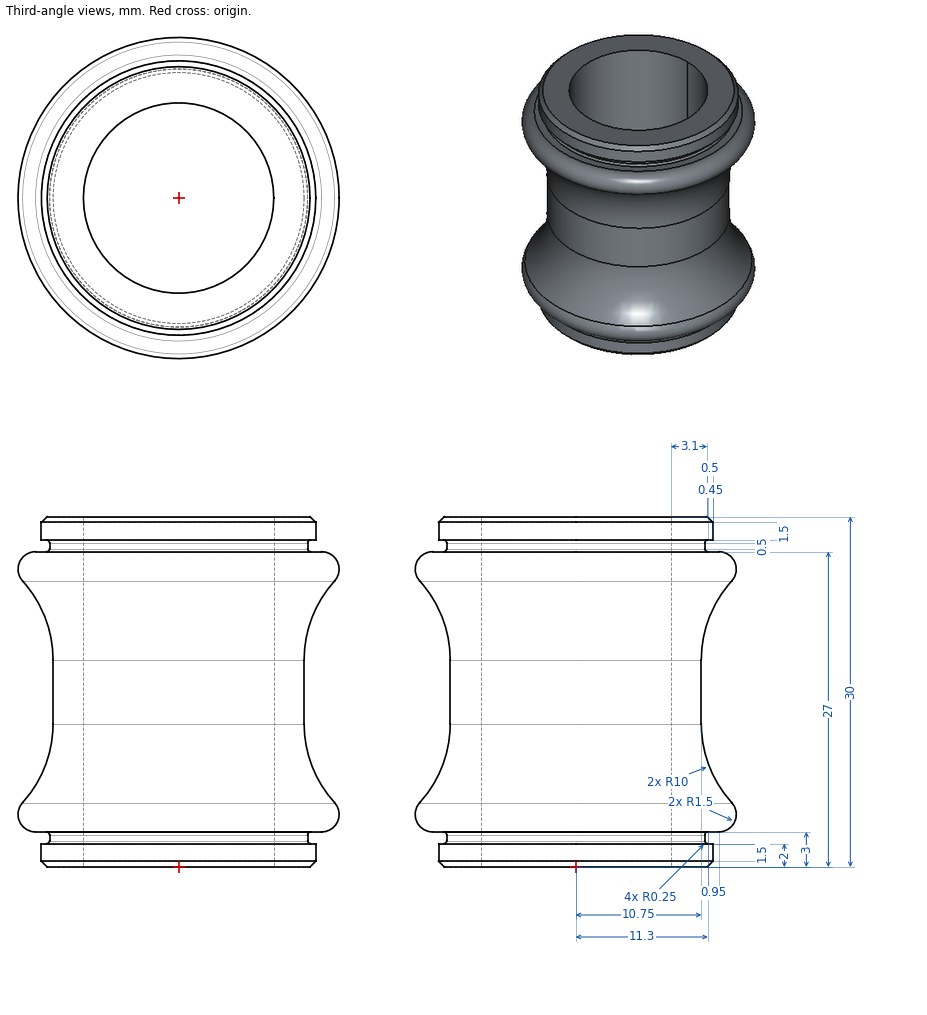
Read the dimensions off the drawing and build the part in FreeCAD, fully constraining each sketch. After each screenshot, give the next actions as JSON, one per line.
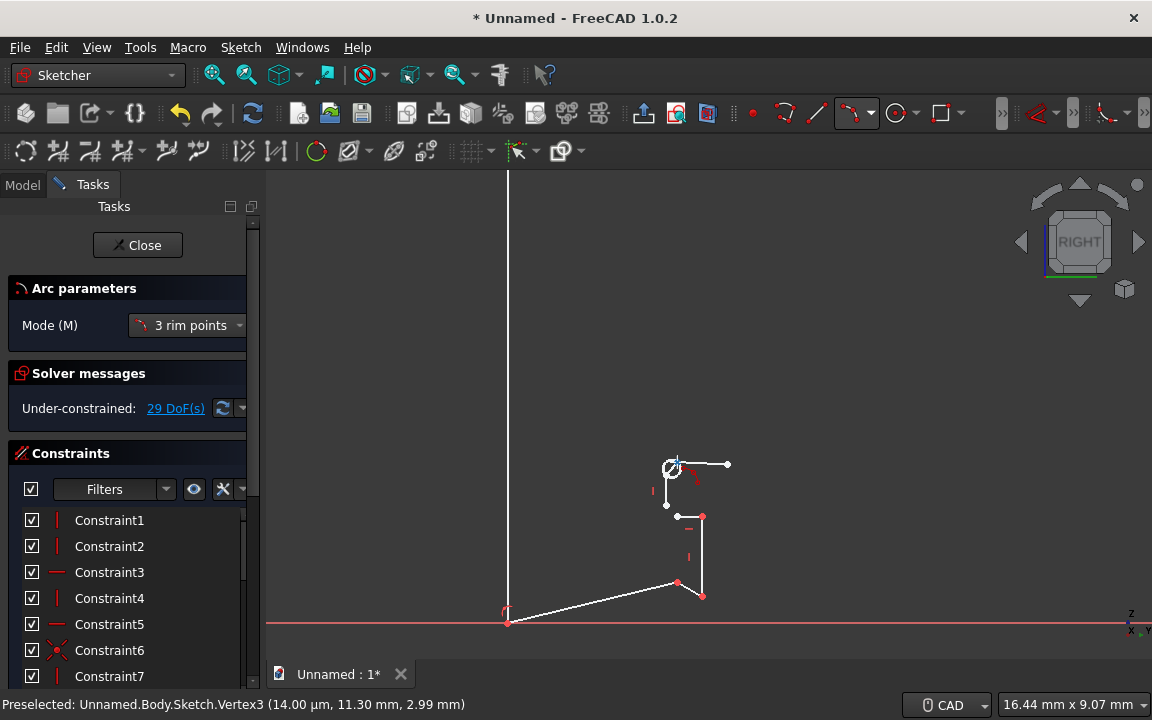
{"action": "scroll", "coordinate": [668, 465], "scroll_direction": "up", "scroll_amount": 7}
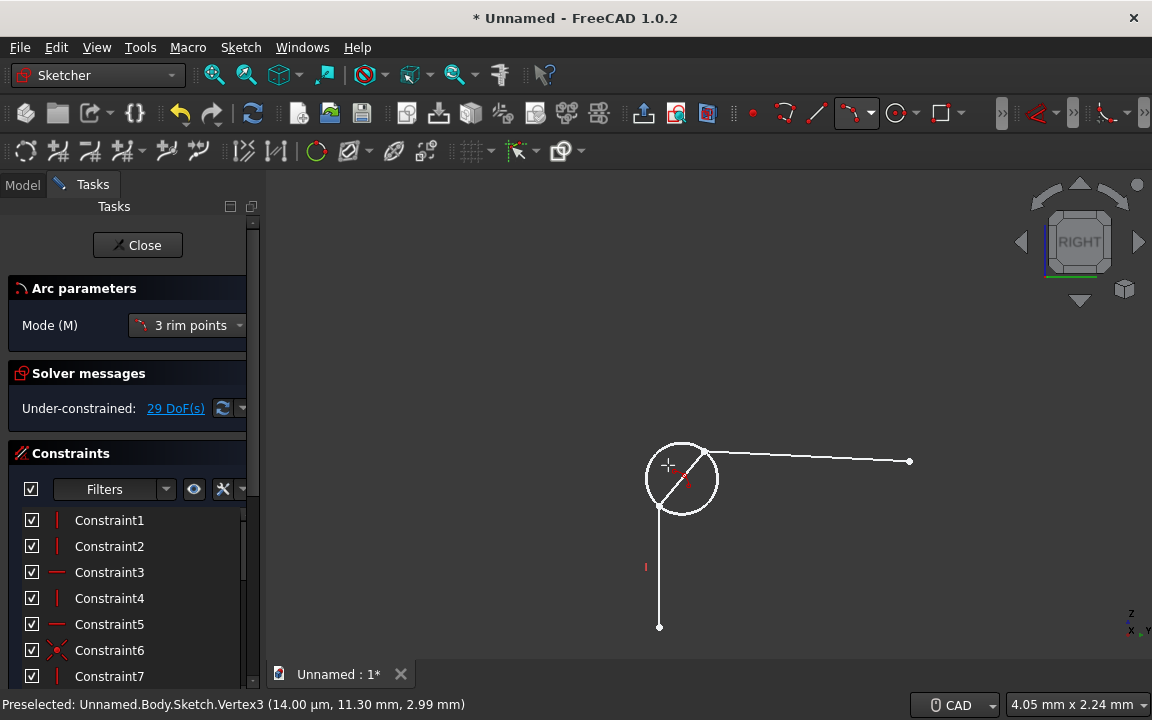
{"action": "left_click", "coordinate": [667, 464]}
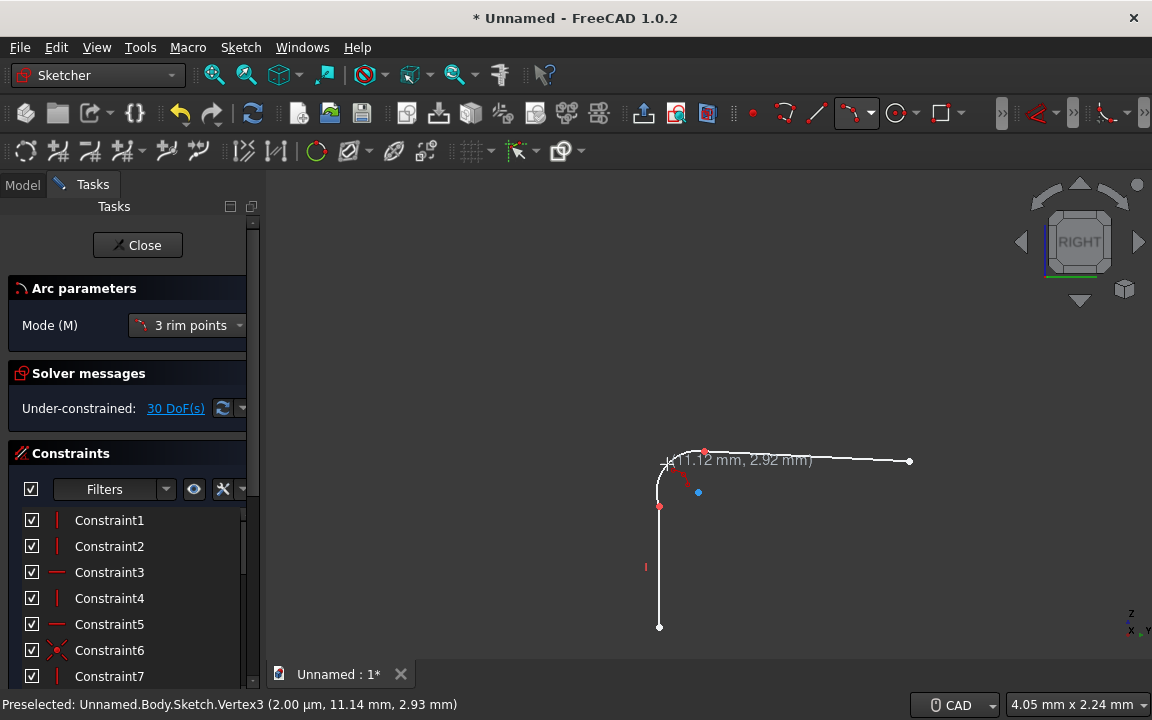
{"action": "scroll", "coordinate": [689, 550], "scroll_direction": "down", "scroll_amount": 15}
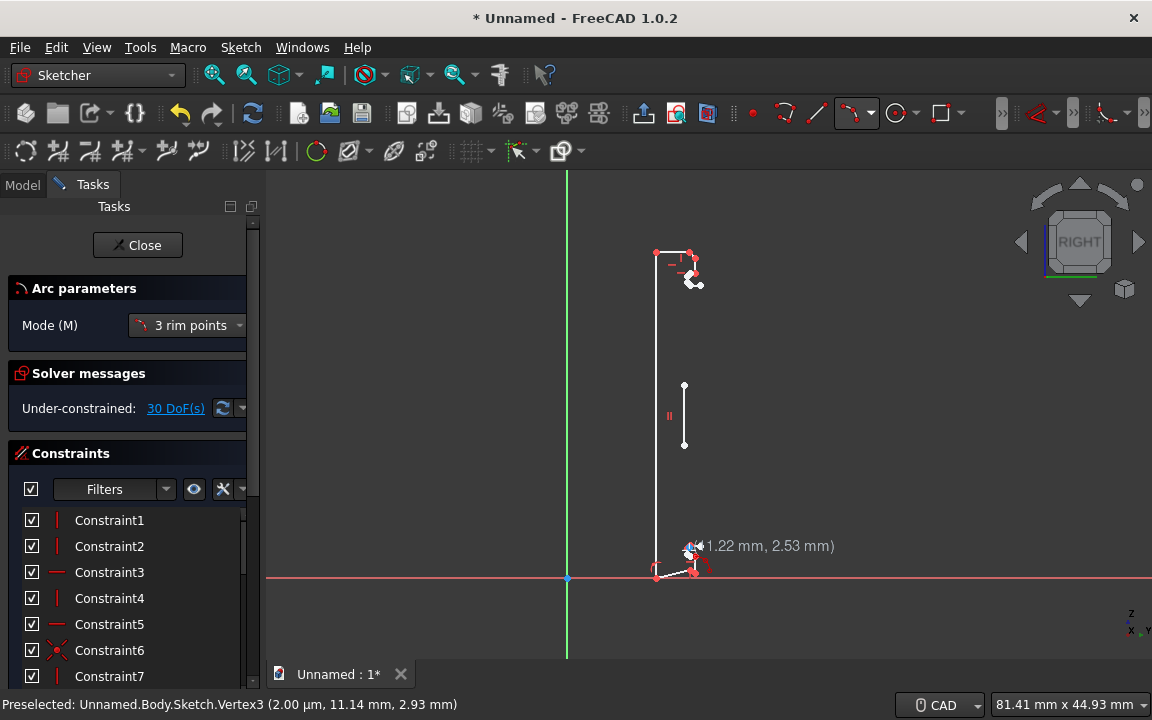
{"action": "scroll", "coordinate": [701, 546], "scroll_direction": "up", "scroll_amount": 6}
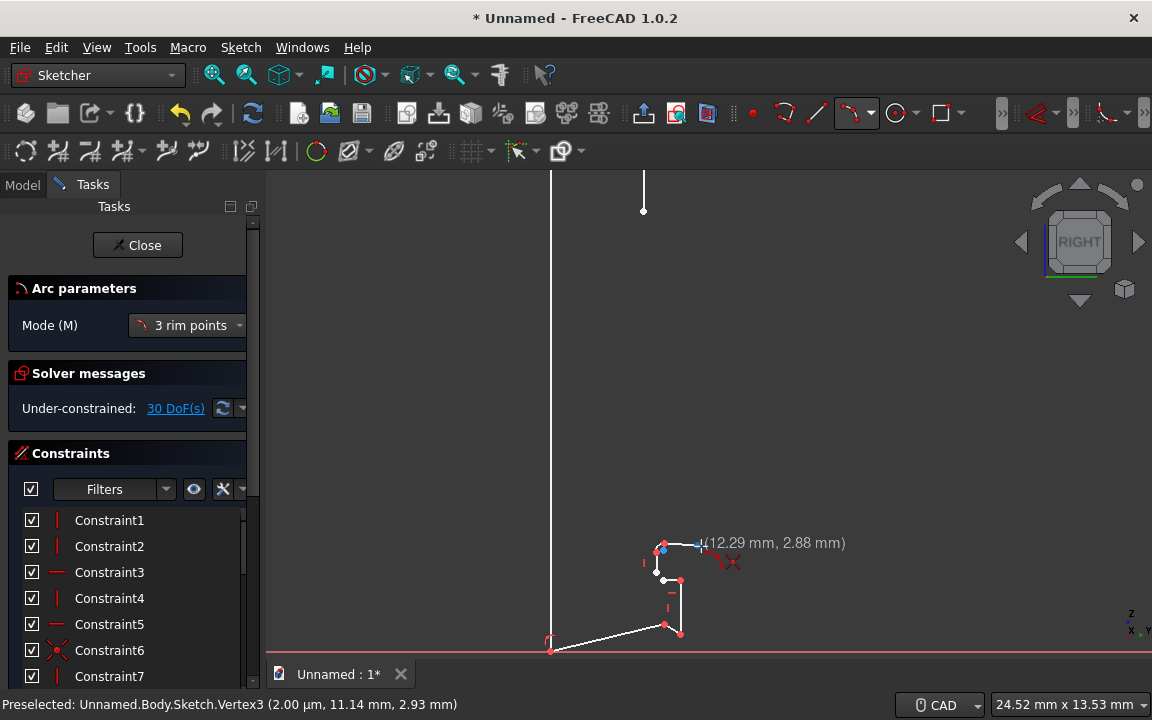
{"action": "left_click", "coordinate": [698, 545]}
{"action": "left_click", "coordinate": [739, 452]}
{"action": "left_click", "coordinate": [748, 511]}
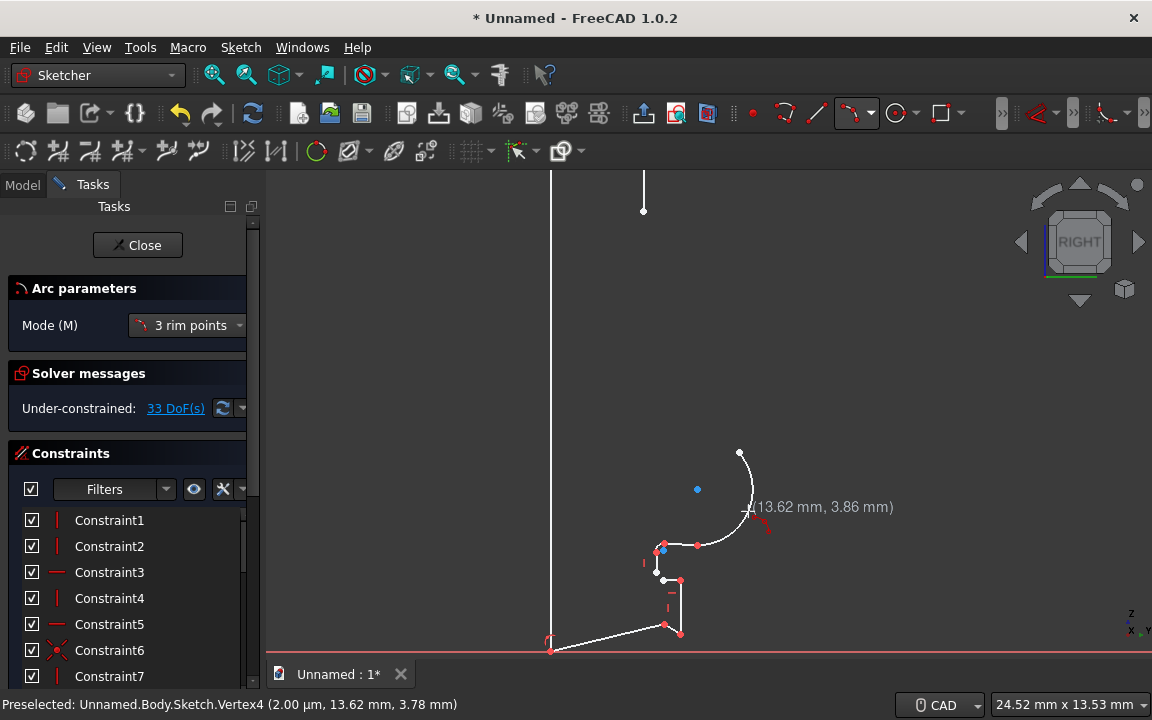
{"action": "left_click", "coordinate": [739, 453]}
{"action": "left_click", "coordinate": [644, 211]}
{"action": "left_click", "coordinate": [669, 340]}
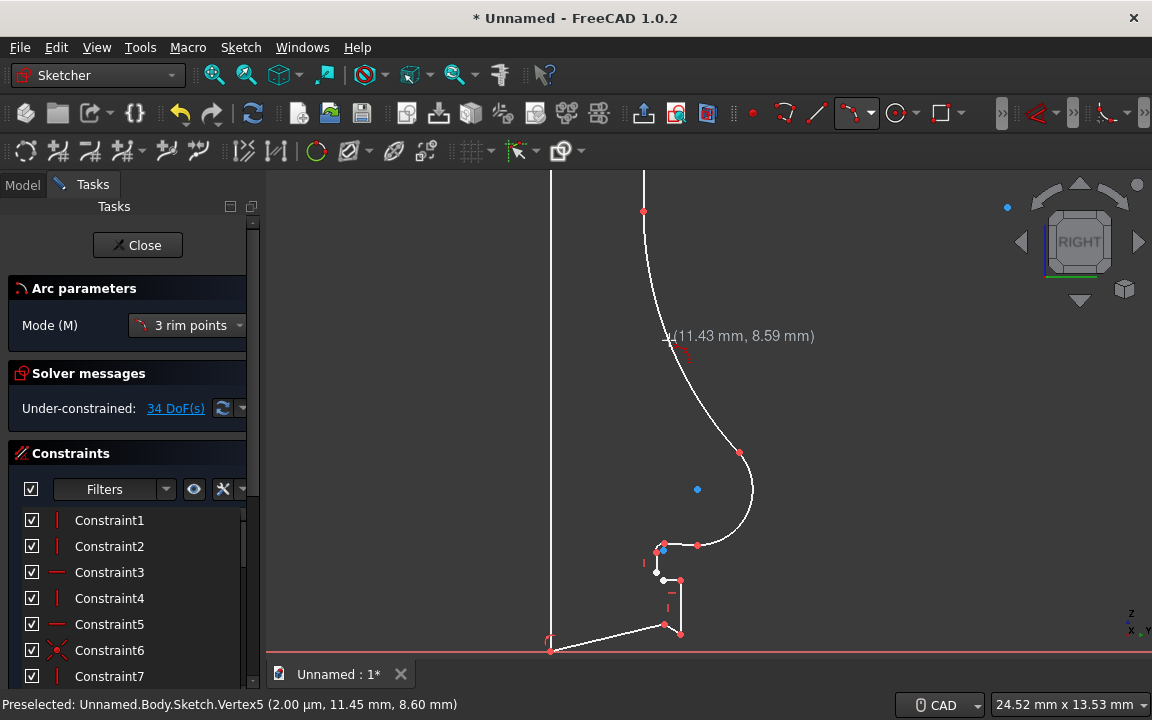
{"action": "scroll", "coordinate": [700, 546], "scroll_direction": "down", "scroll_amount": 6}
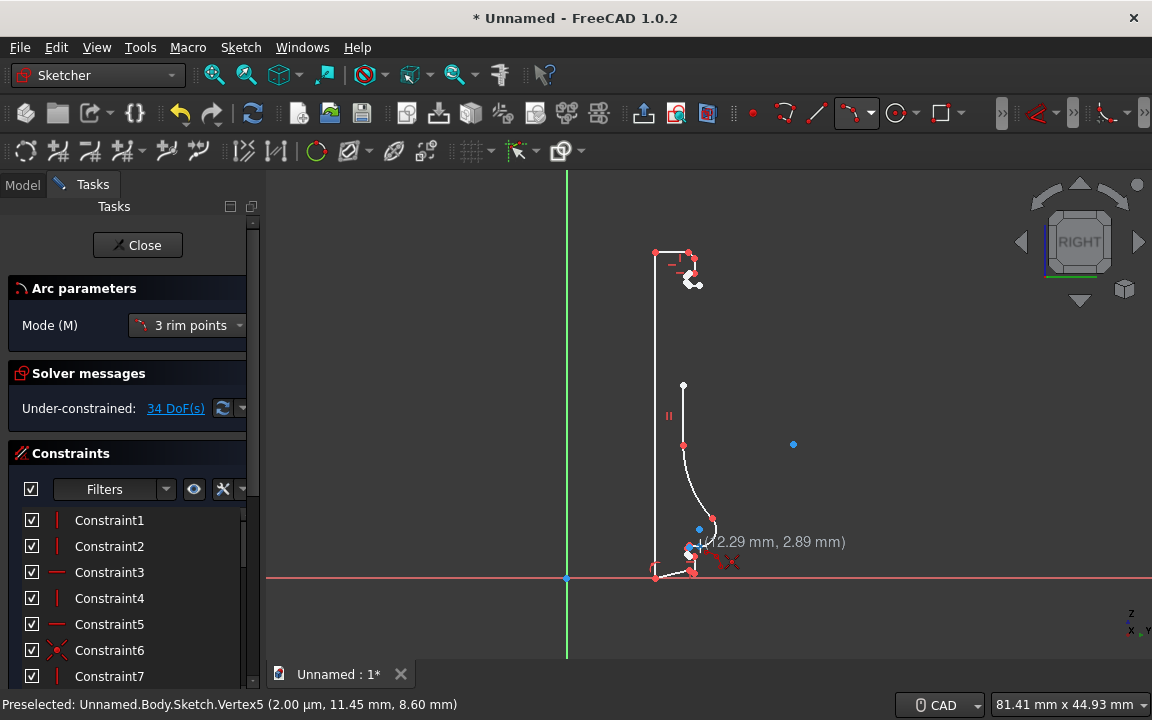
{"action": "left_click", "coordinate": [683, 386]}
{"action": "left_click", "coordinate": [712, 312]}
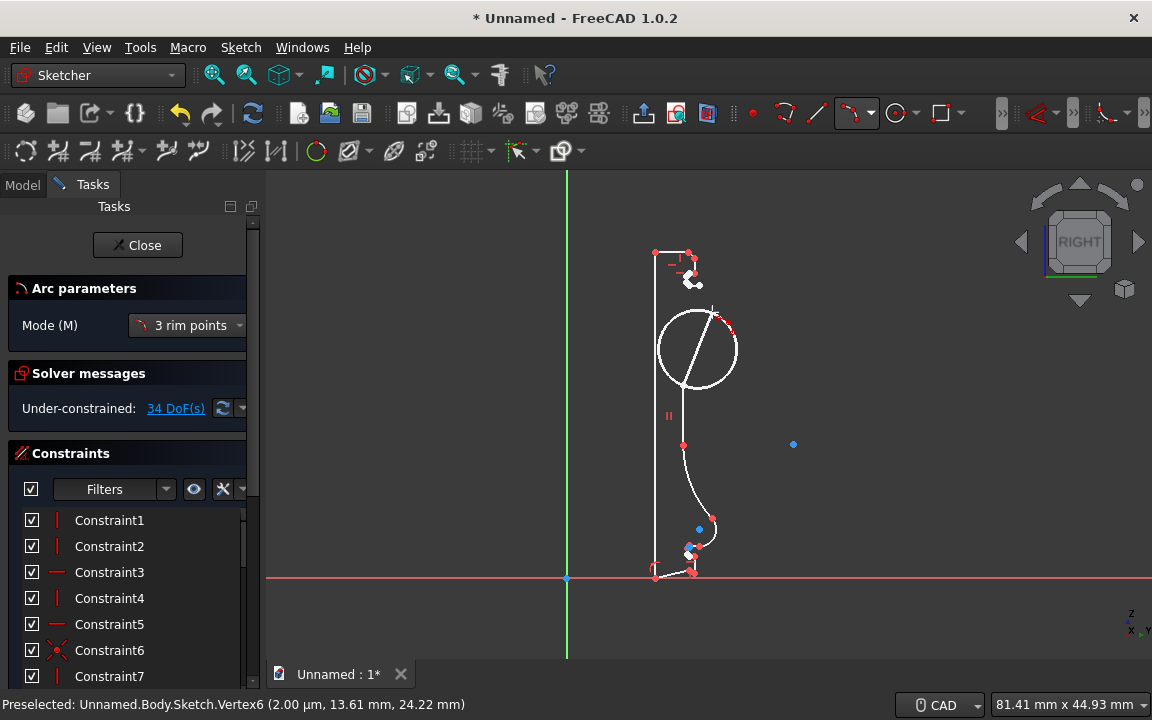
{"action": "scroll", "coordinate": [691, 346], "scroll_direction": "up", "scroll_amount": 4}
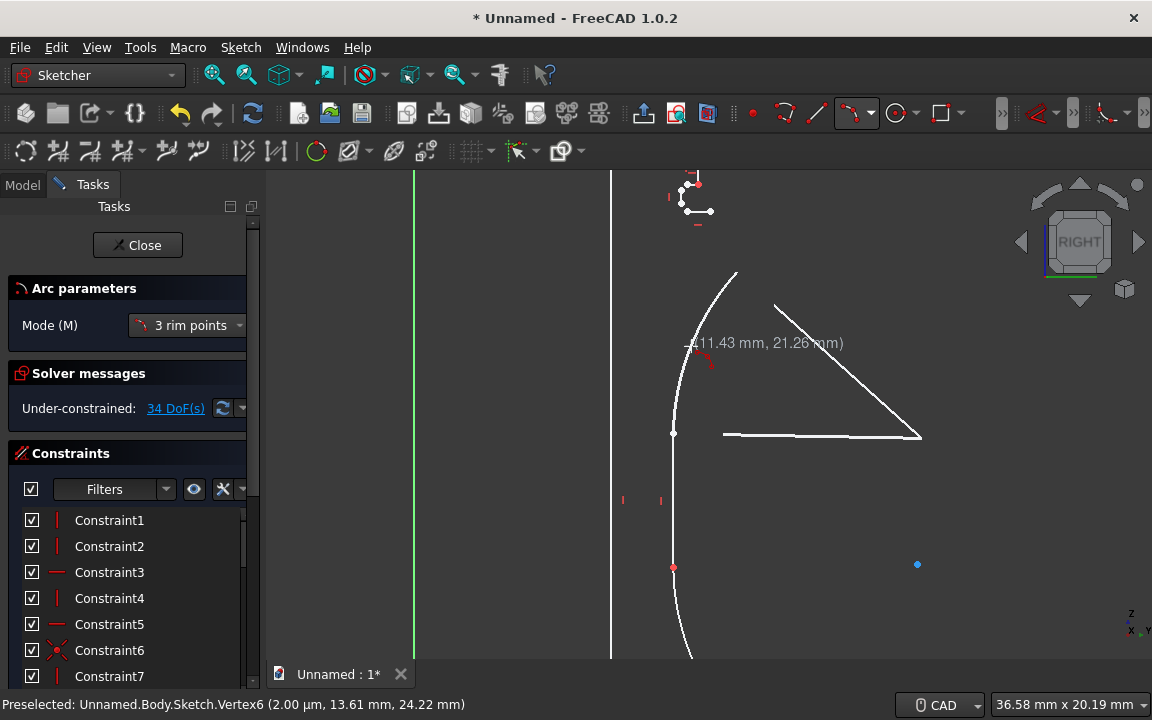
{"action": "left_click", "coordinate": [690, 345]}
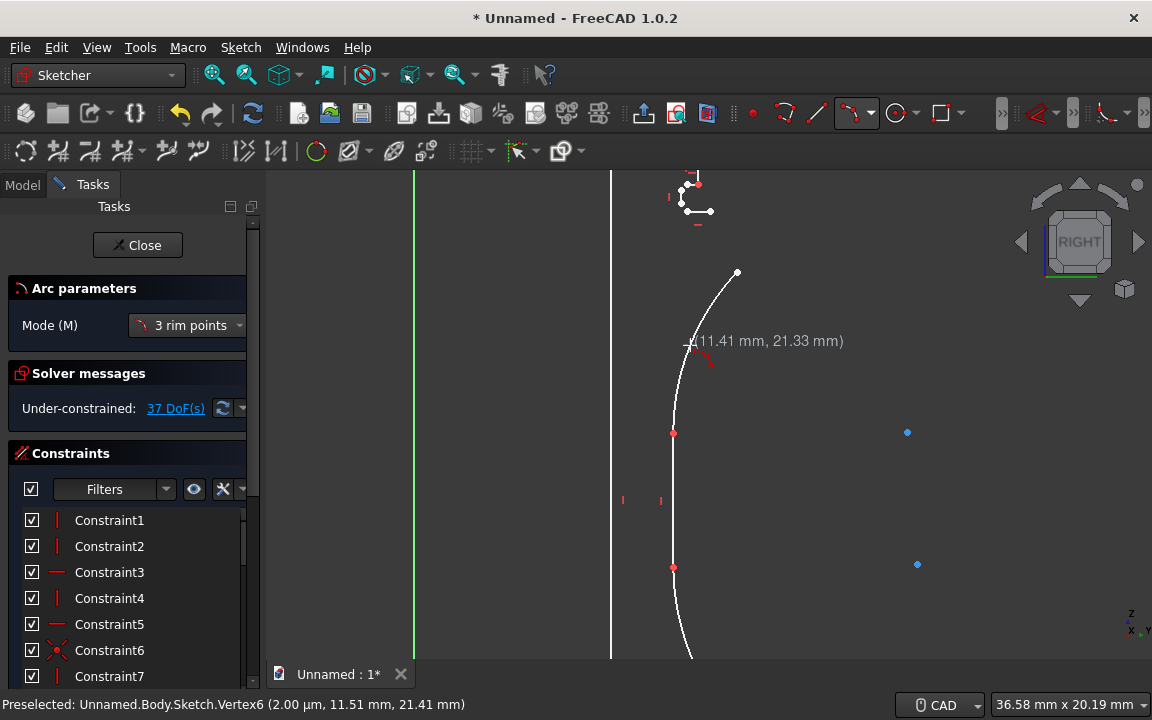
{"action": "left_click", "coordinate": [737, 272]}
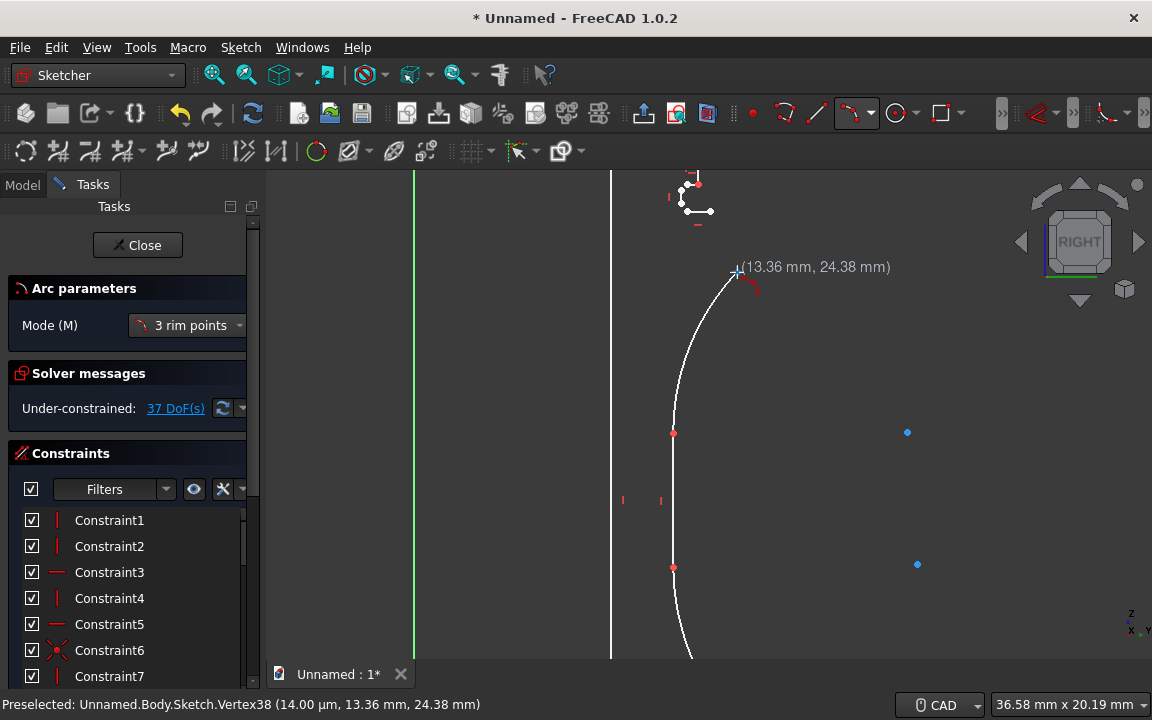
{"action": "scroll", "coordinate": [710, 209], "scroll_direction": "up", "scroll_amount": 2}